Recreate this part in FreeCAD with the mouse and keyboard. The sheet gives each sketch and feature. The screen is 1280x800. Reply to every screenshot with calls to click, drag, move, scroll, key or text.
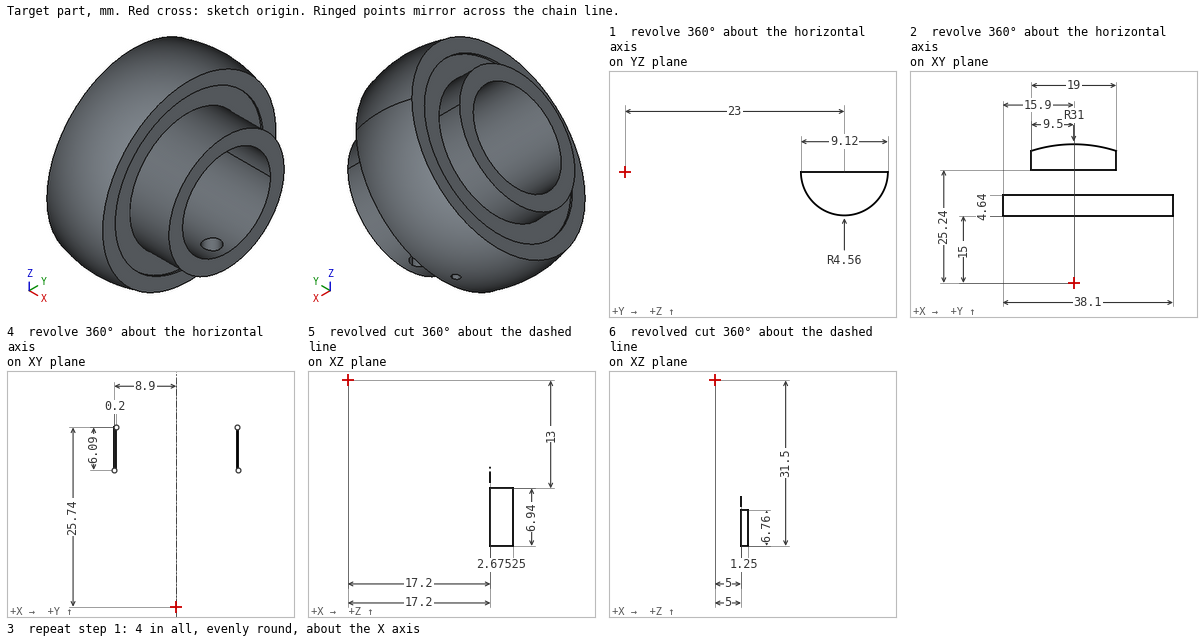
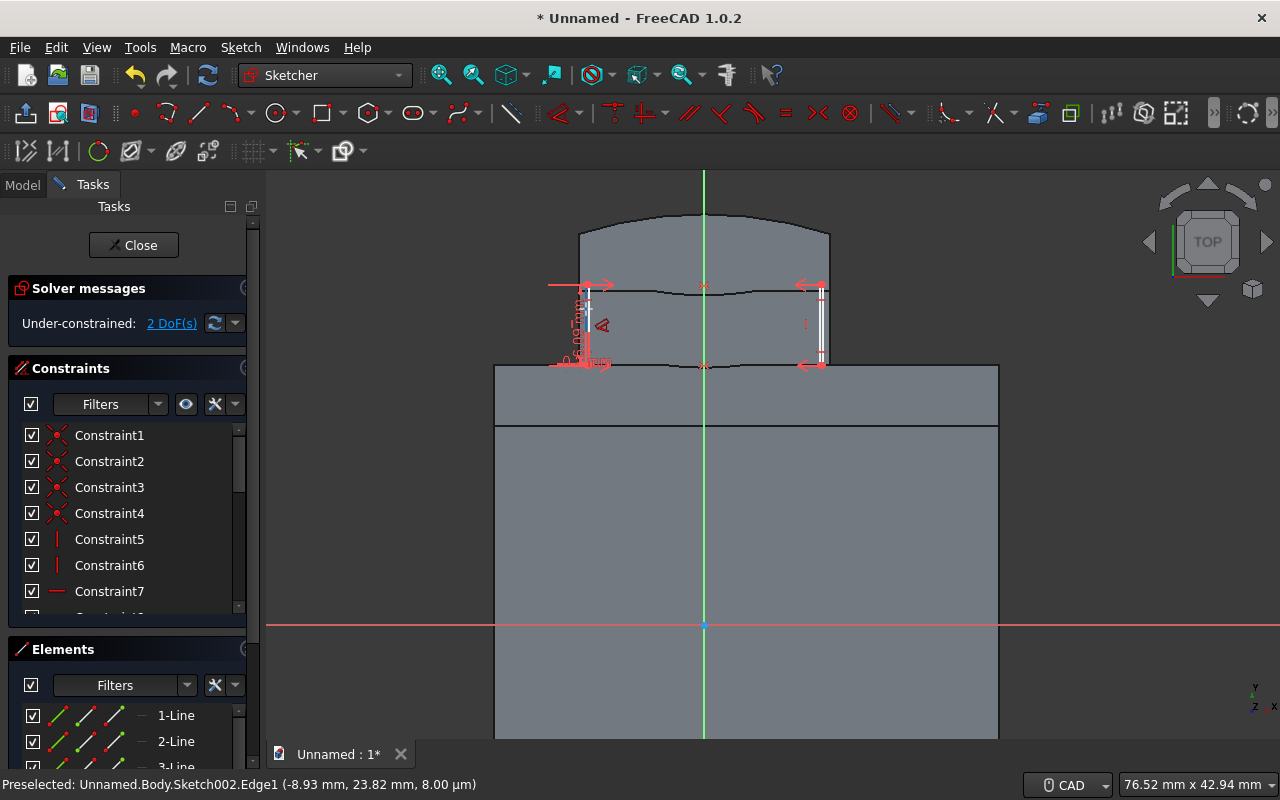
scroll(586, 285, up, 8)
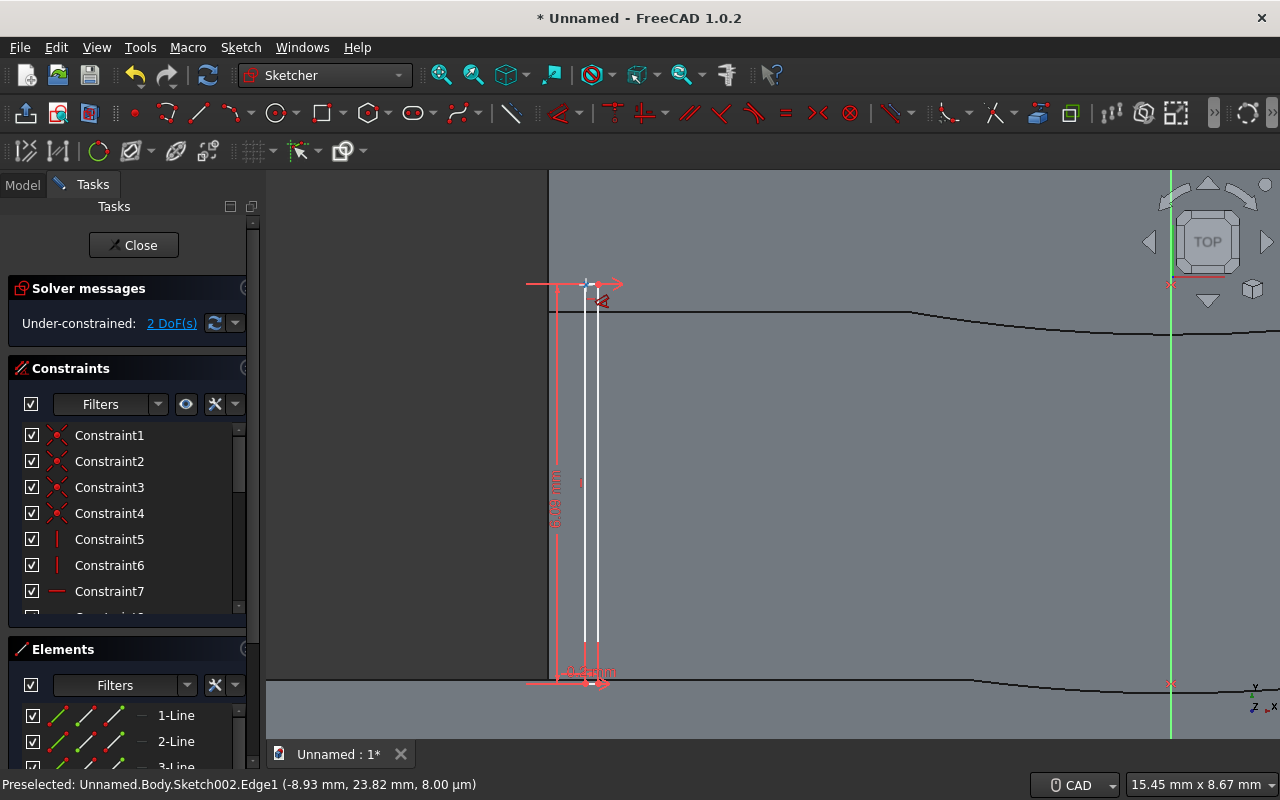
click(585, 284)
click(850, 250)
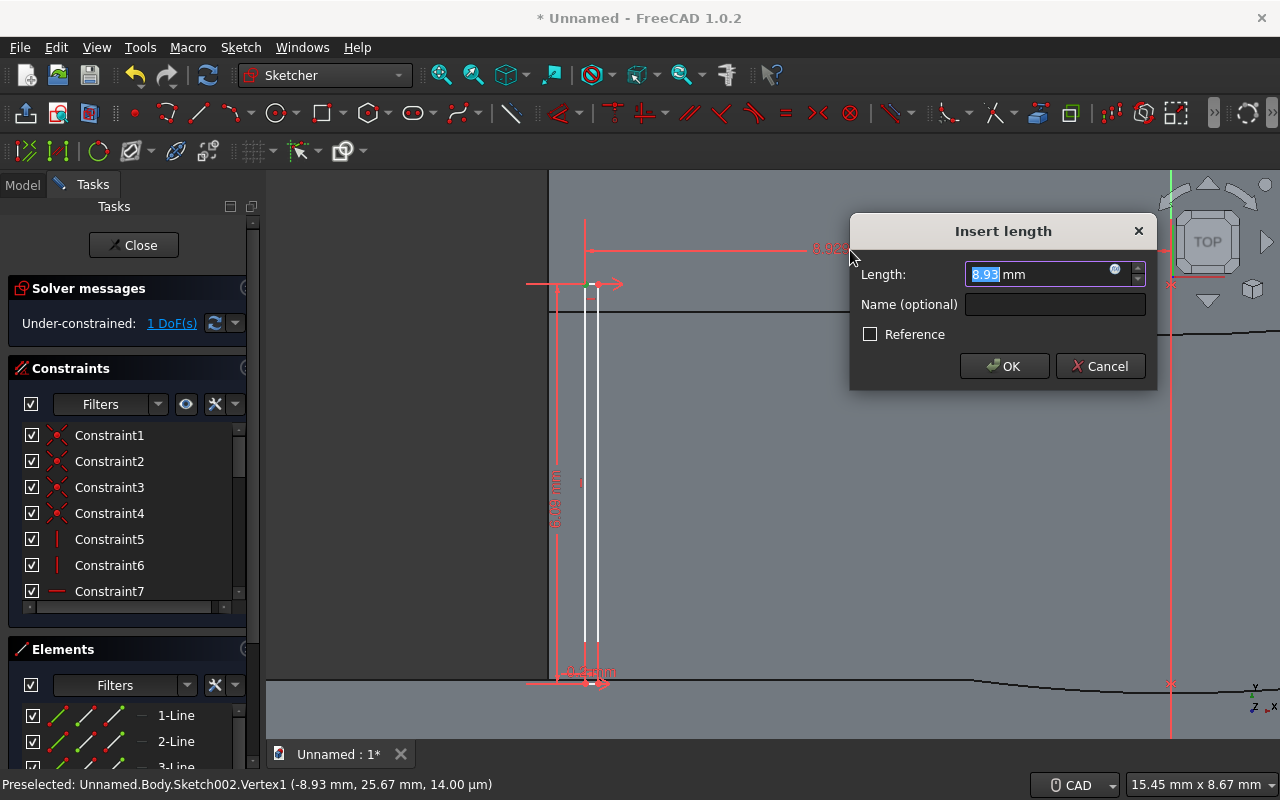
text(8.9)
key(Return)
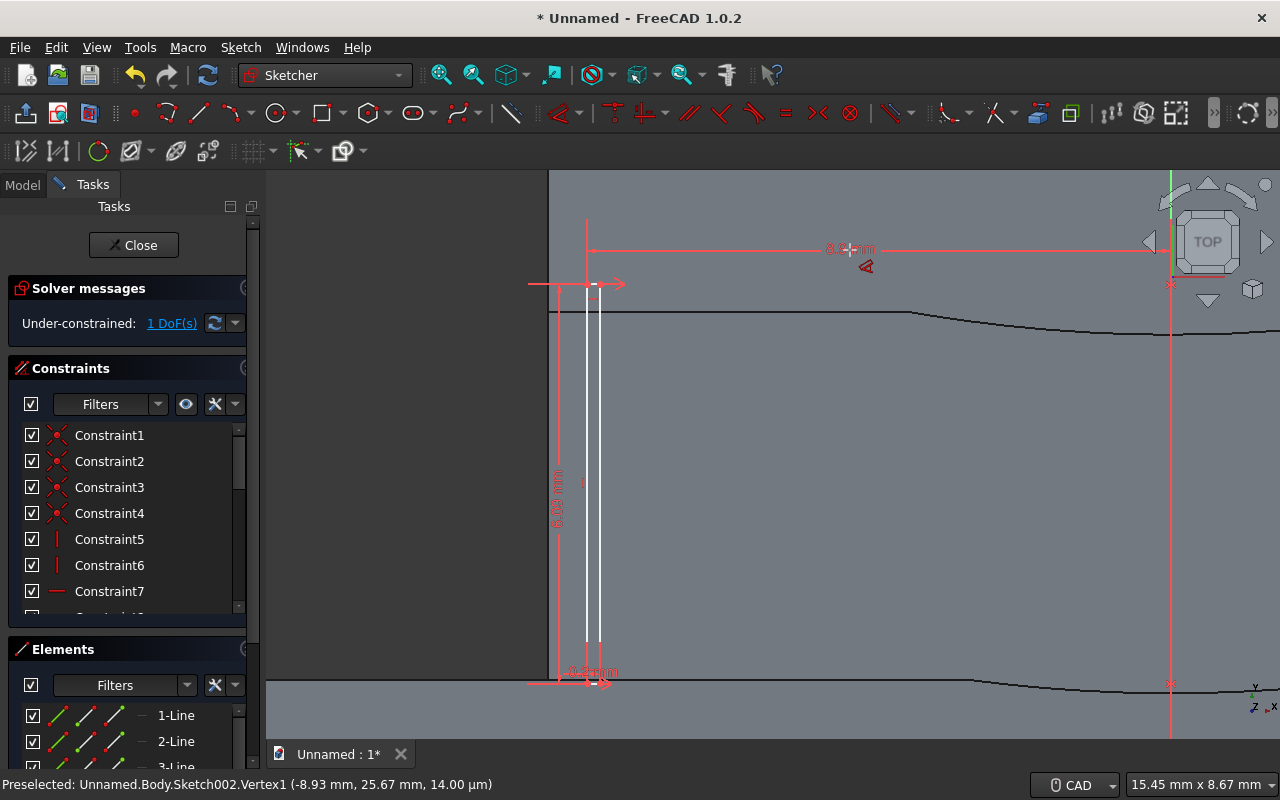
click(587, 284)
click(553, 399)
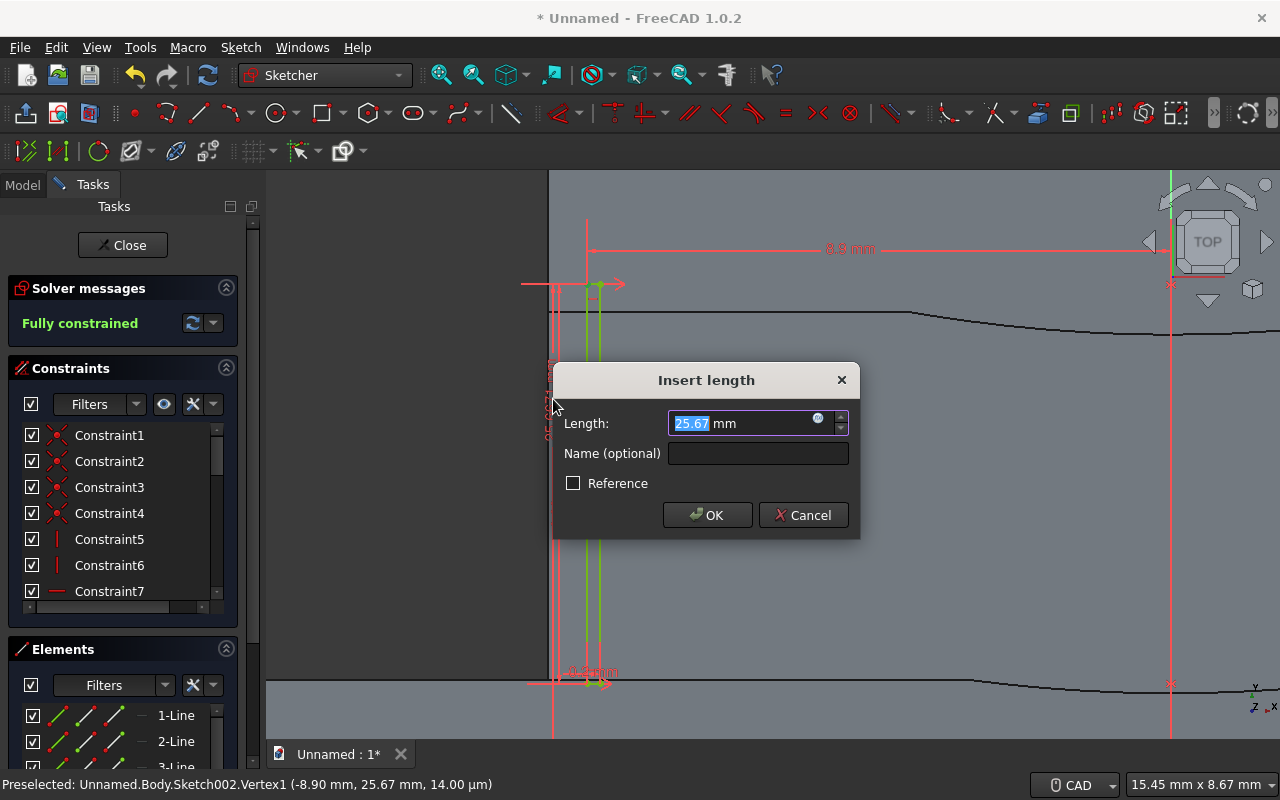
text(25.74)
key(Return)
key(Escape)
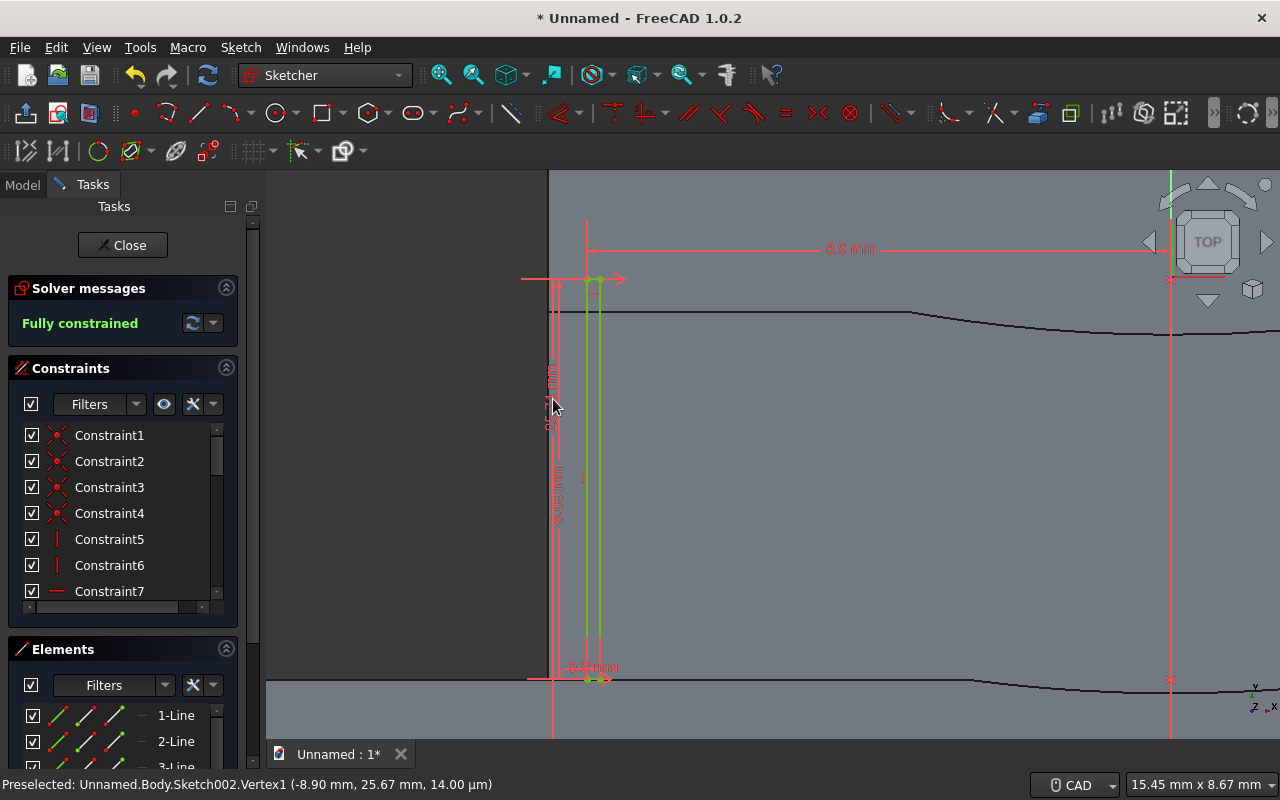
click(123, 245)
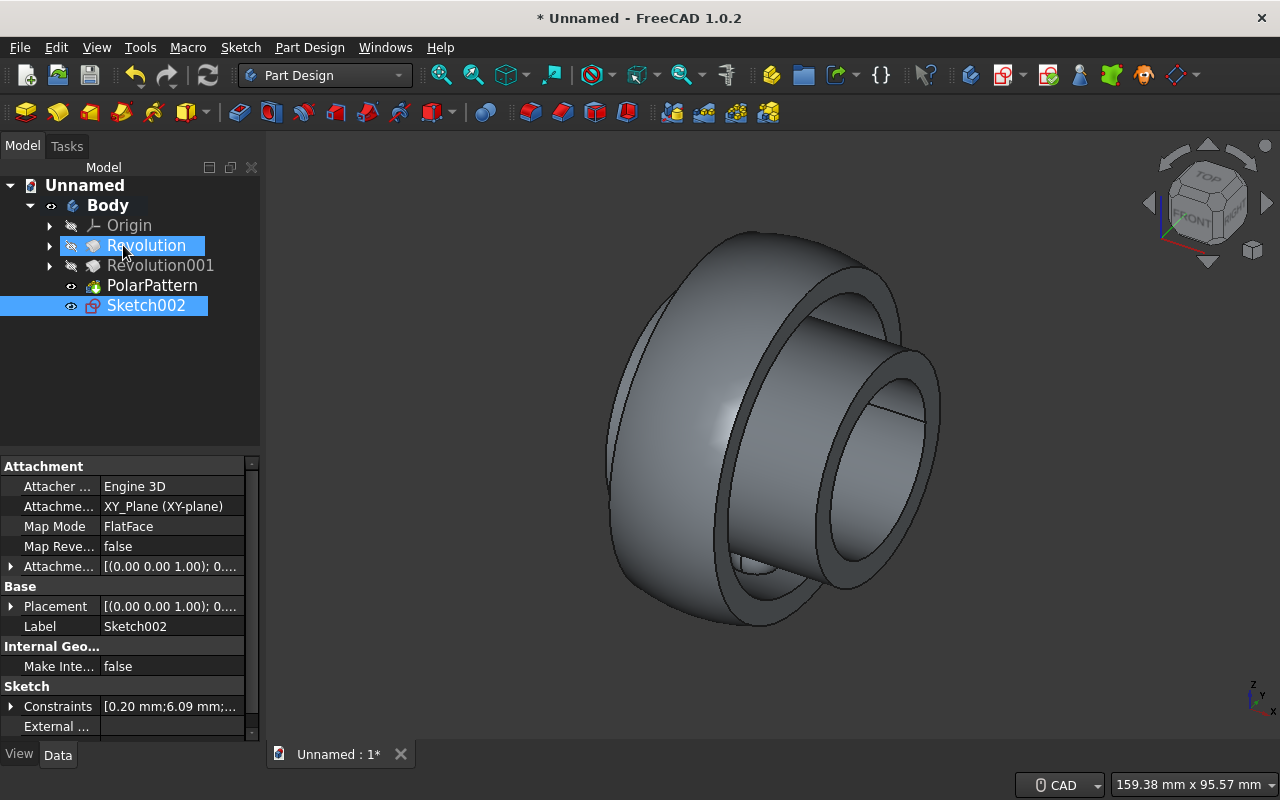
click(58, 112)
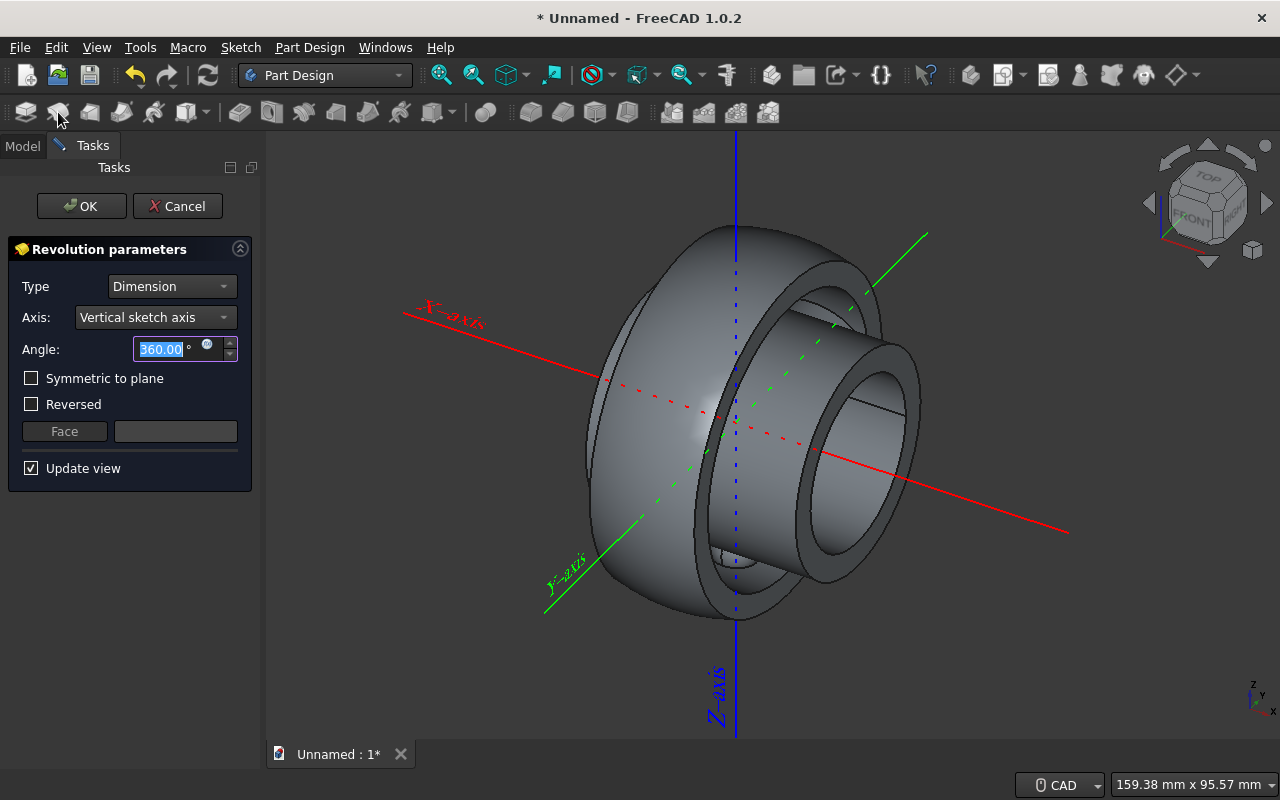
click(156, 318)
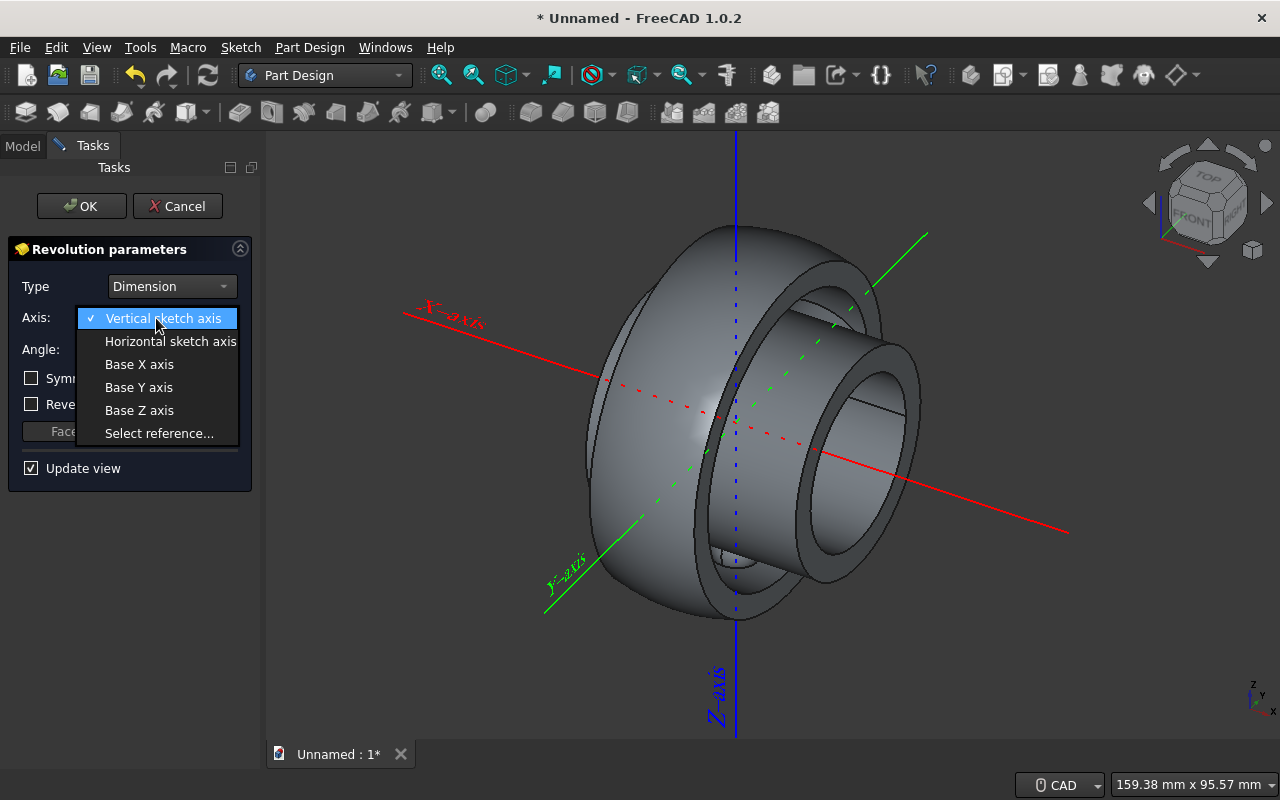
click(156, 342)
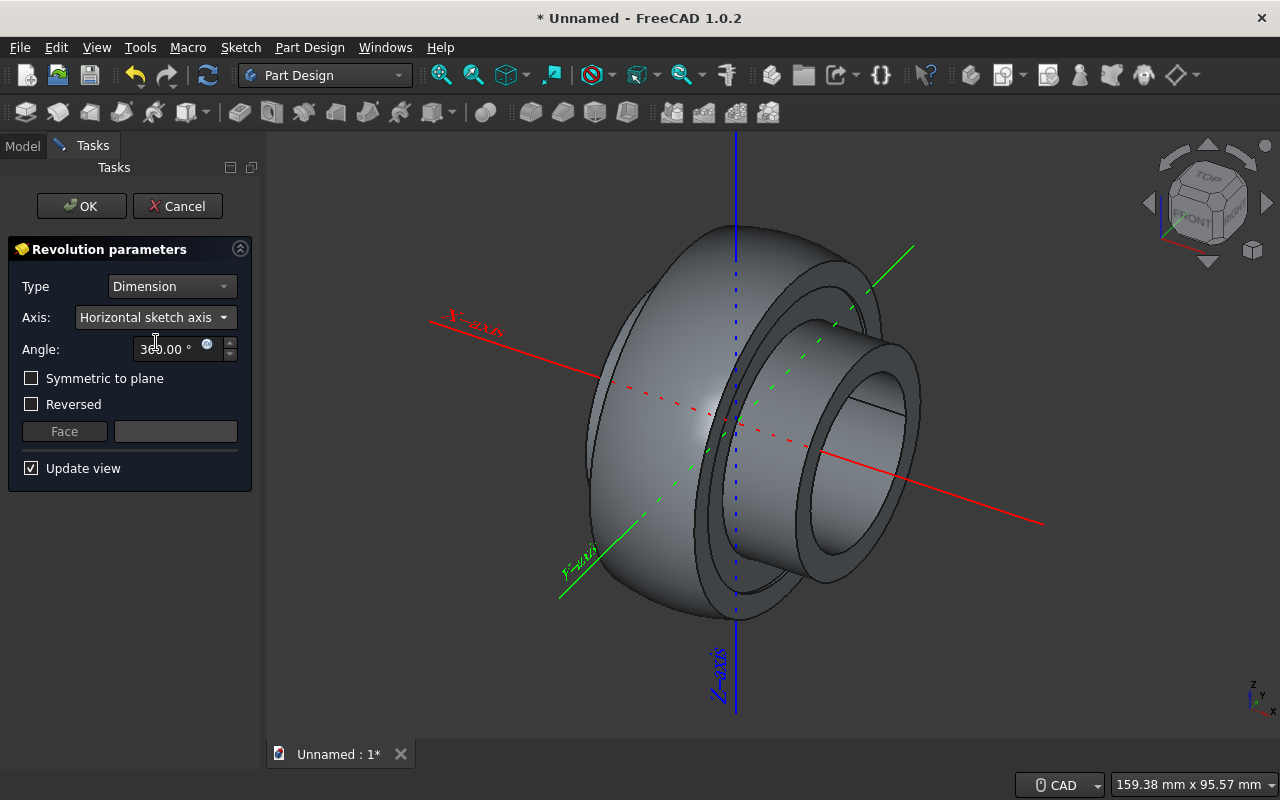
click(82, 206)